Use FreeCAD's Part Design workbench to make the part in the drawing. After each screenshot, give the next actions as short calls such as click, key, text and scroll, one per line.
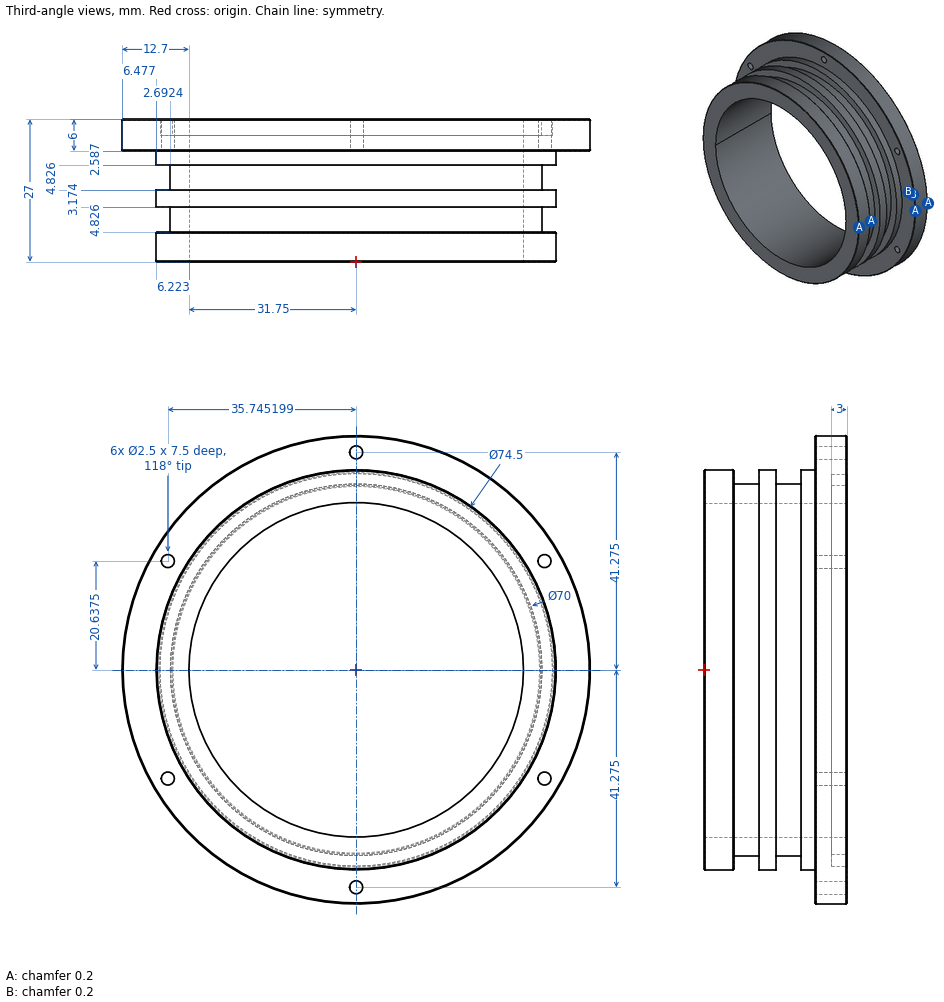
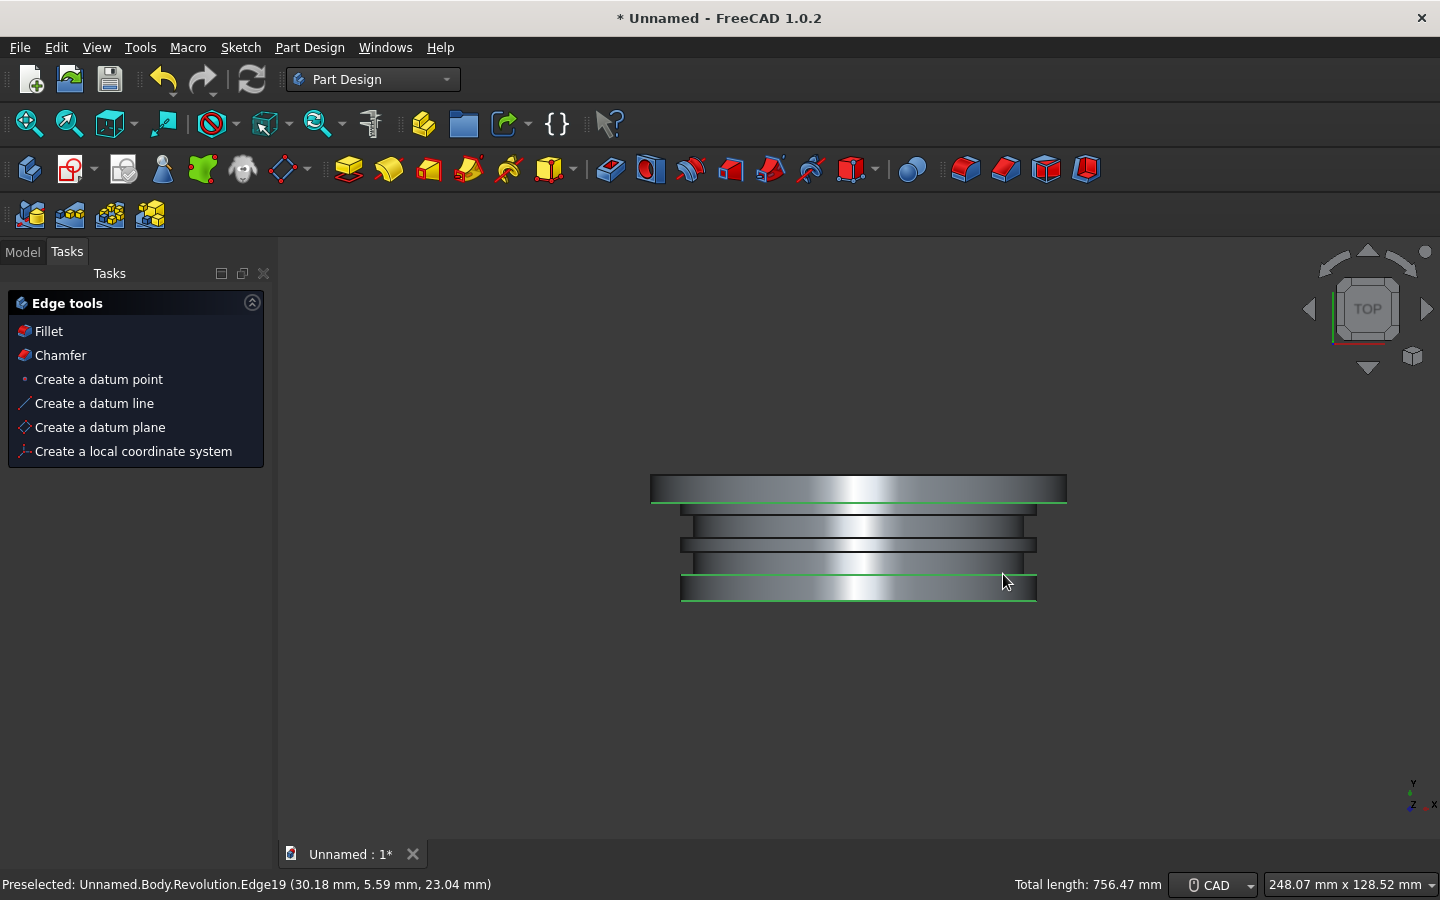
click(1028, 474, ctrl)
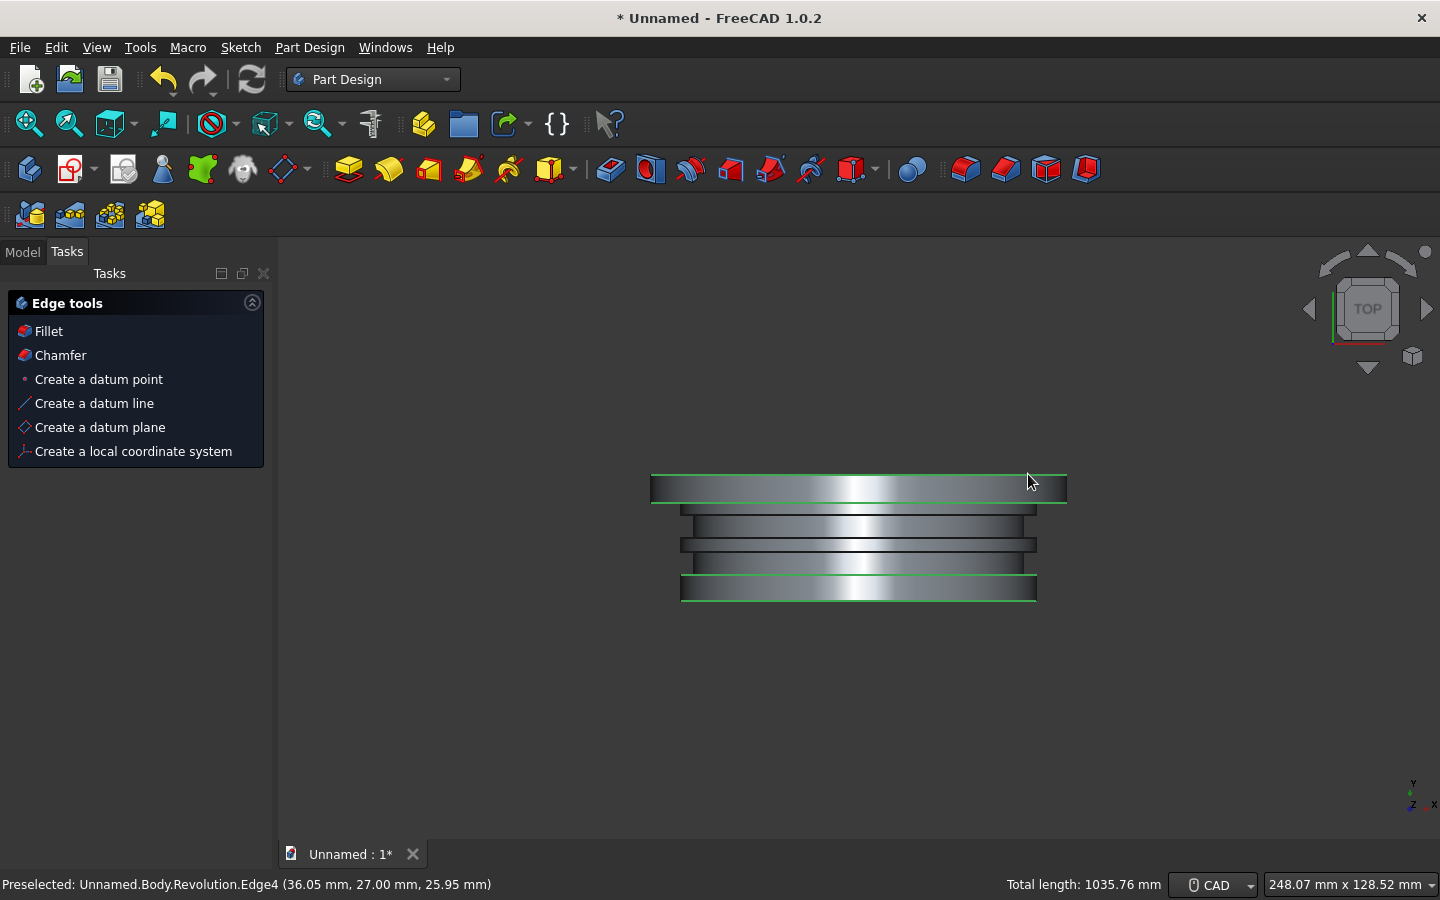
click(1006, 170)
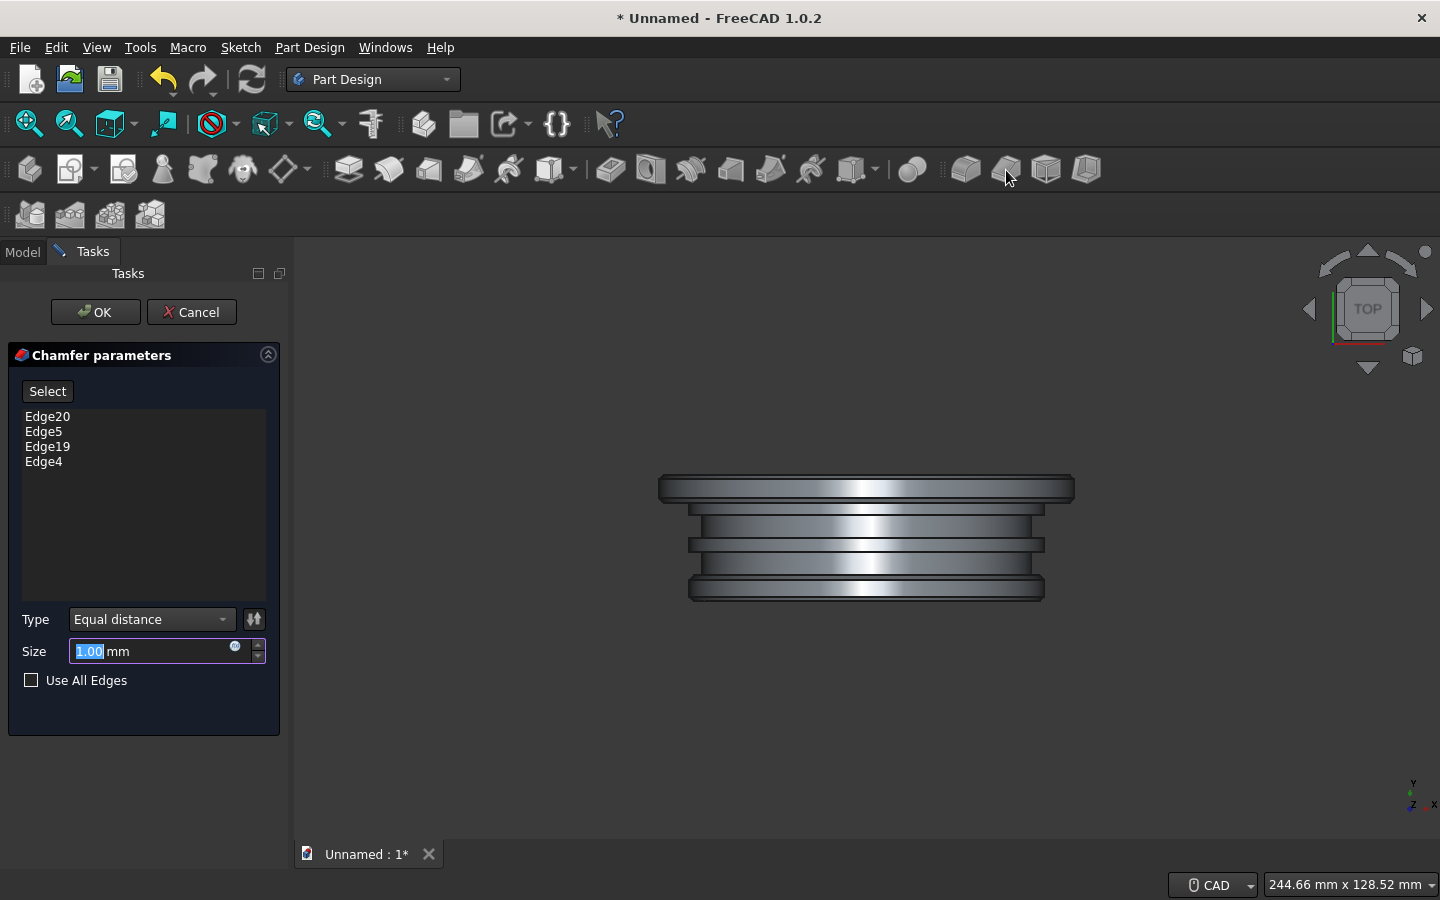
text(0.2)
key(Tab)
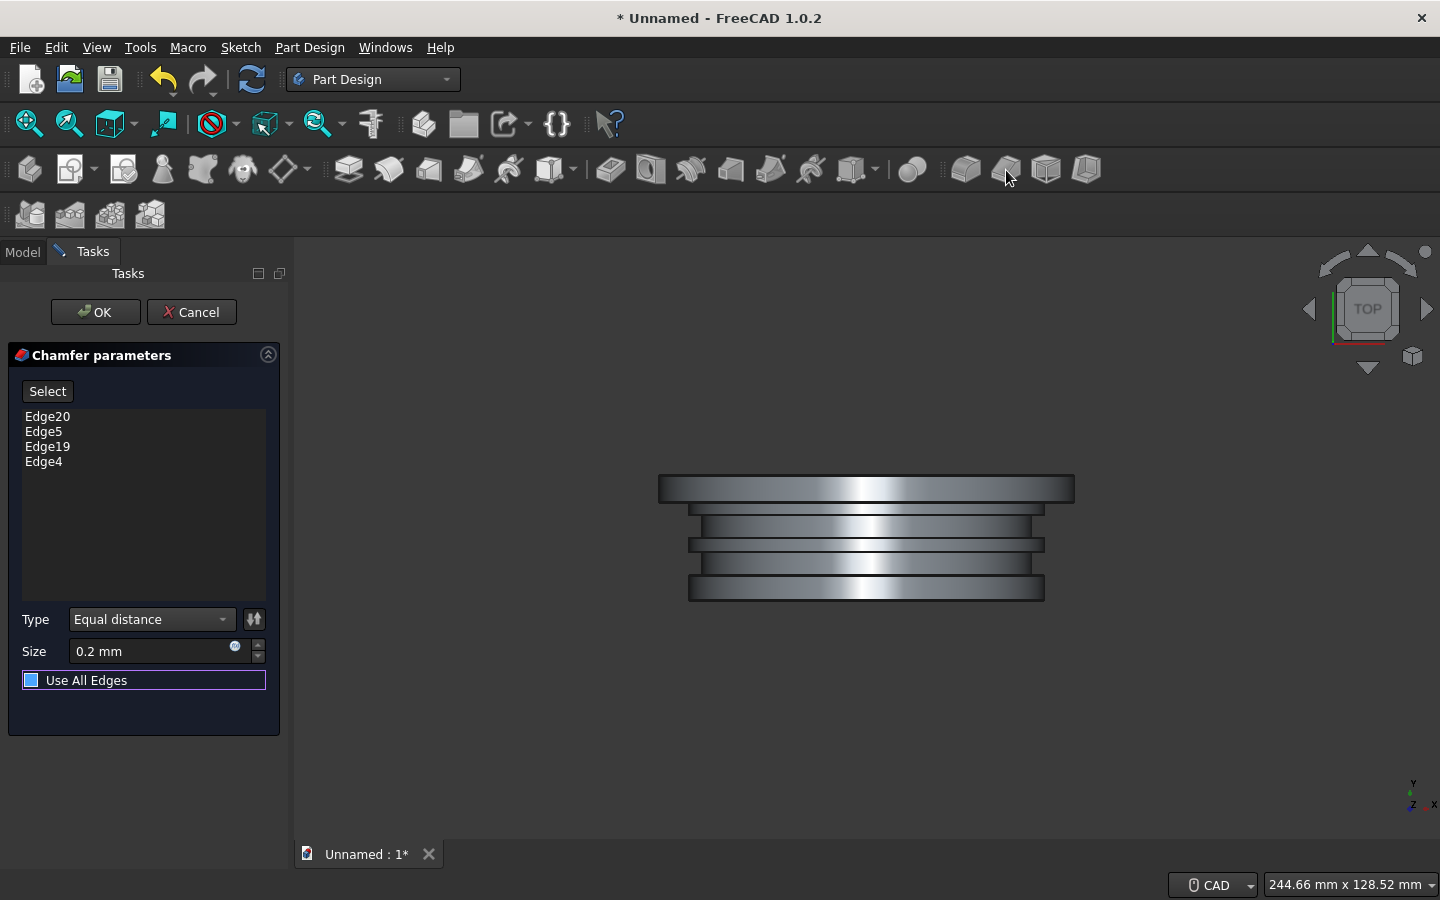
click(96, 312)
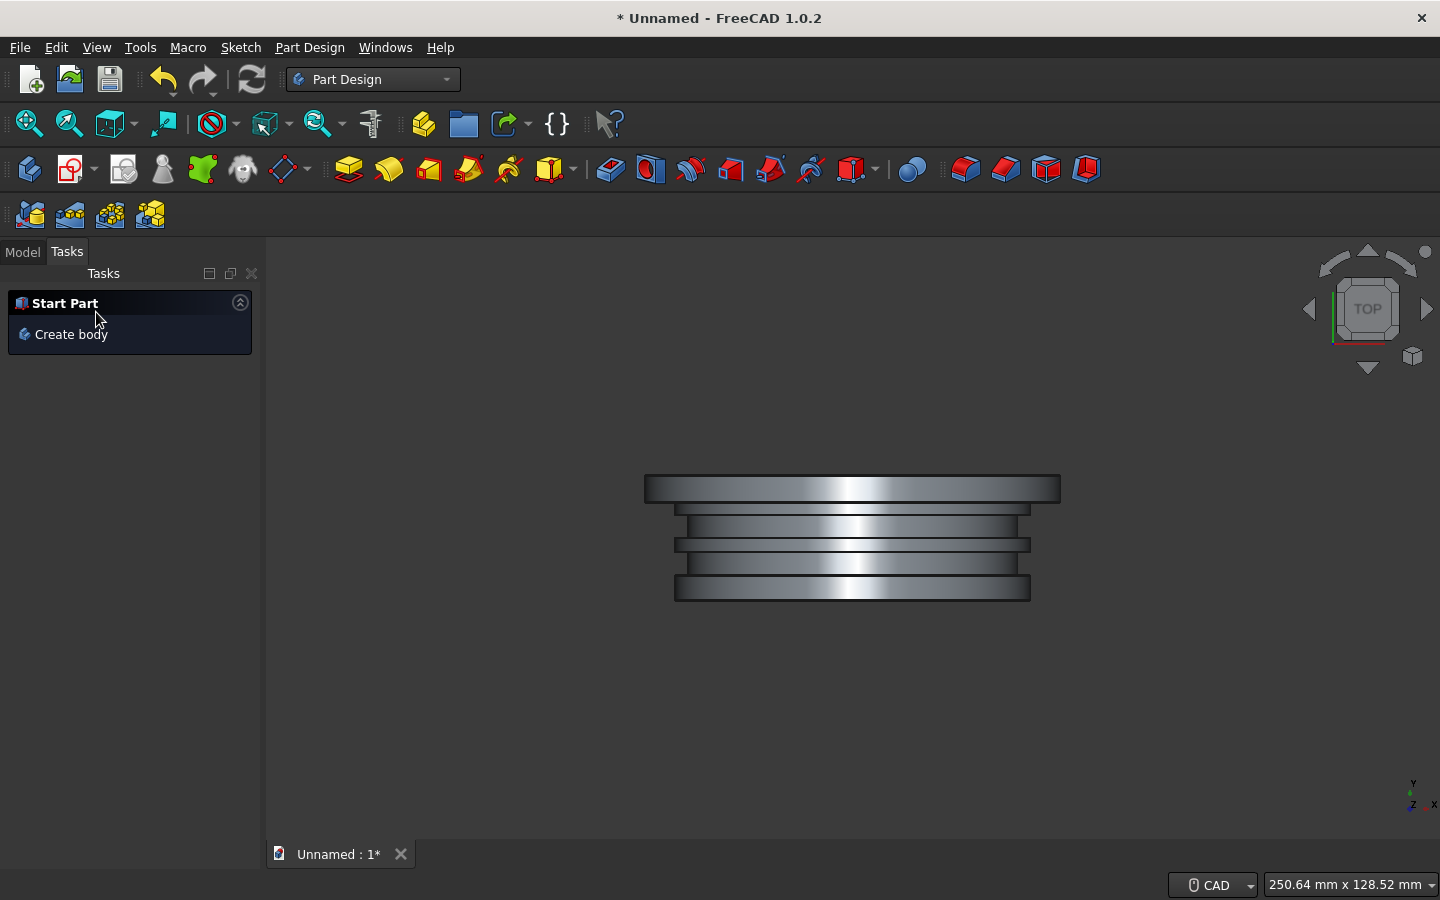
key(v)
key(f)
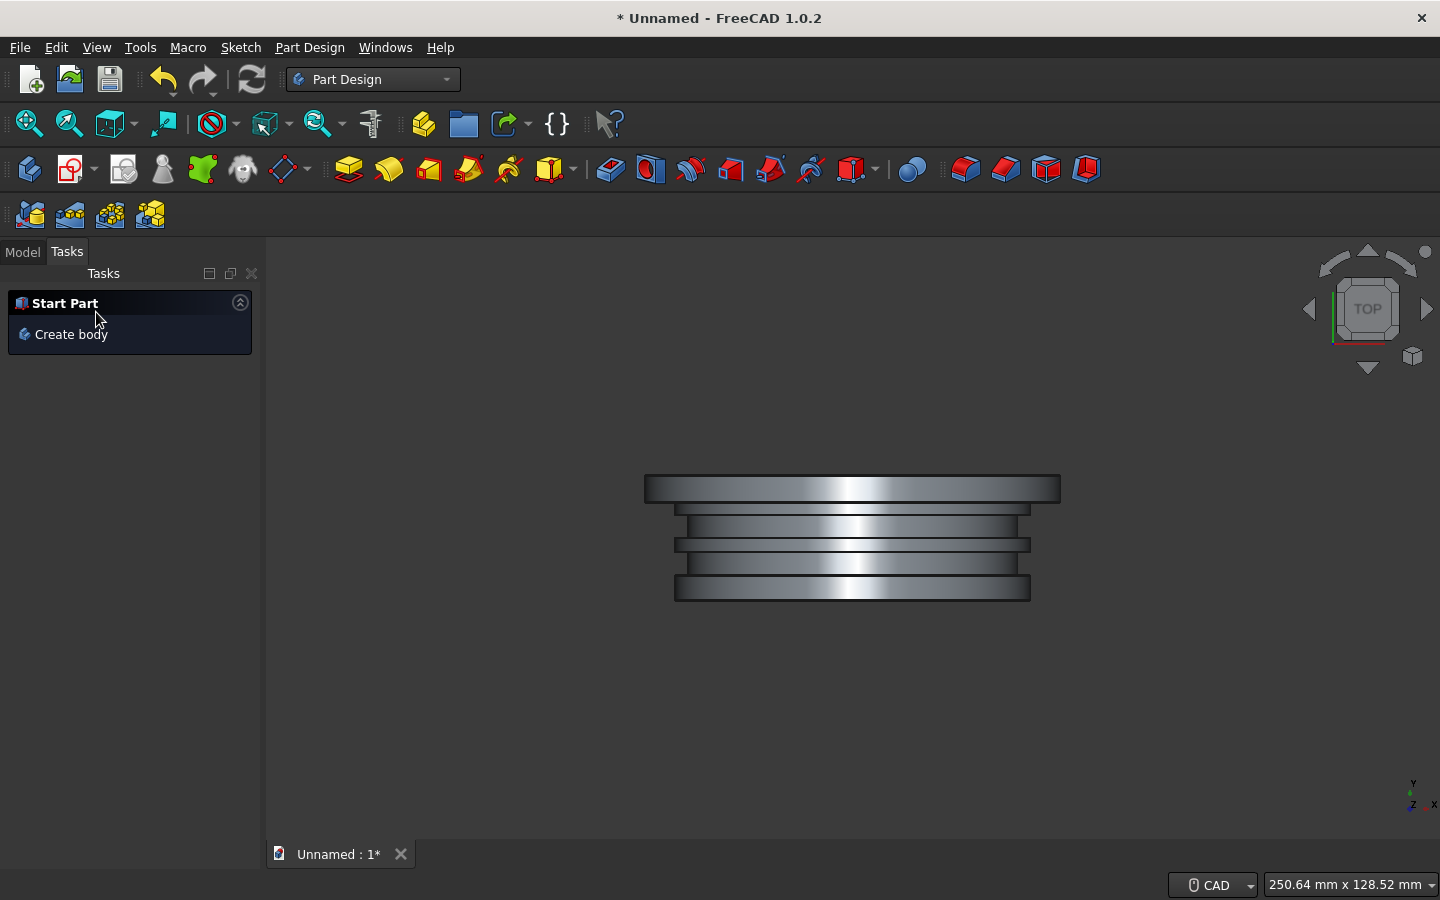
key(4)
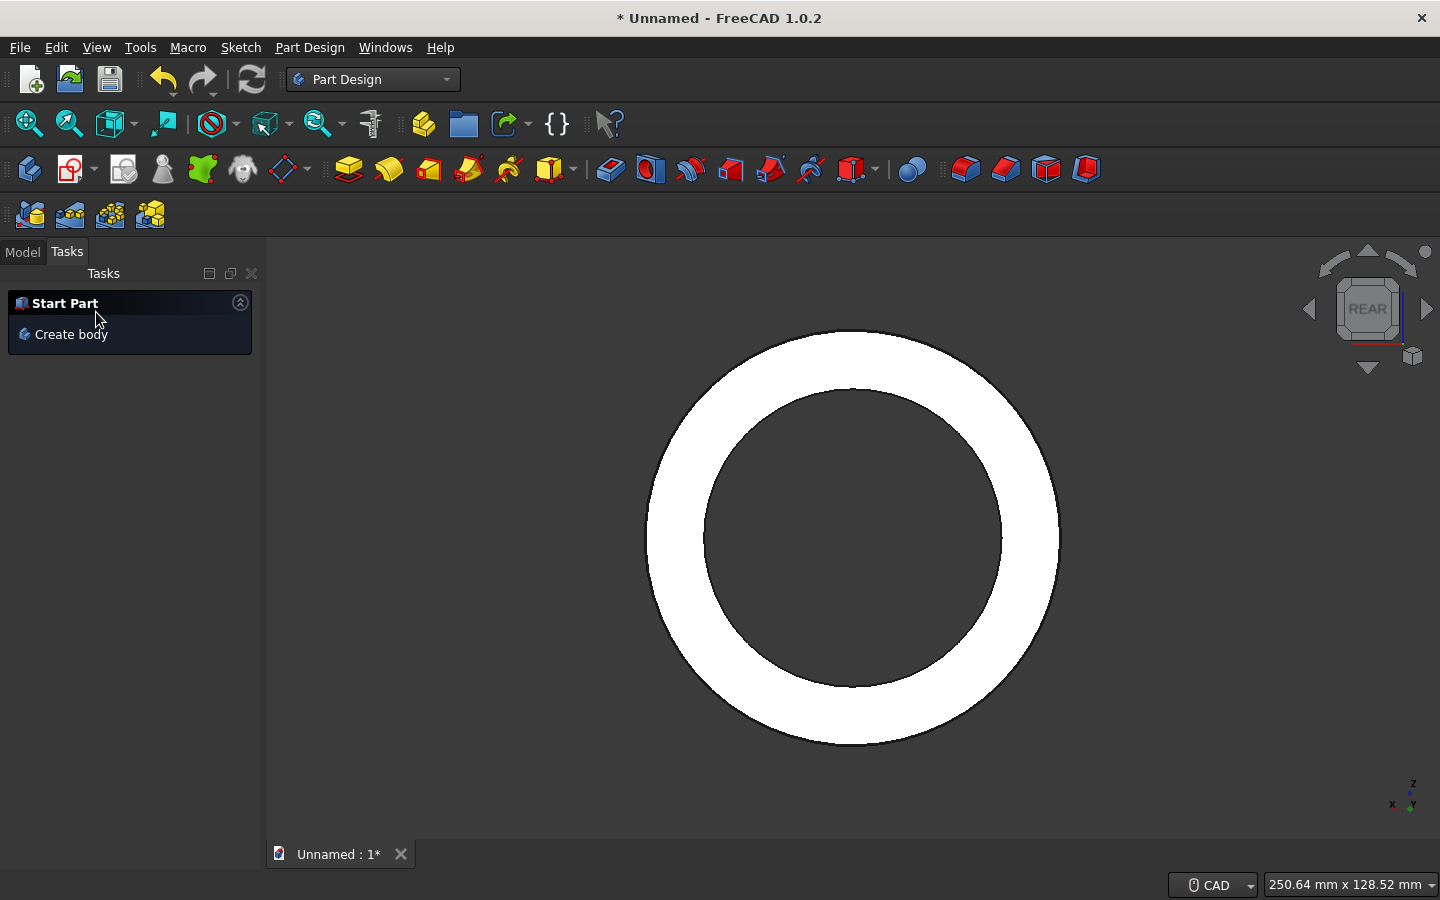
click(675, 537)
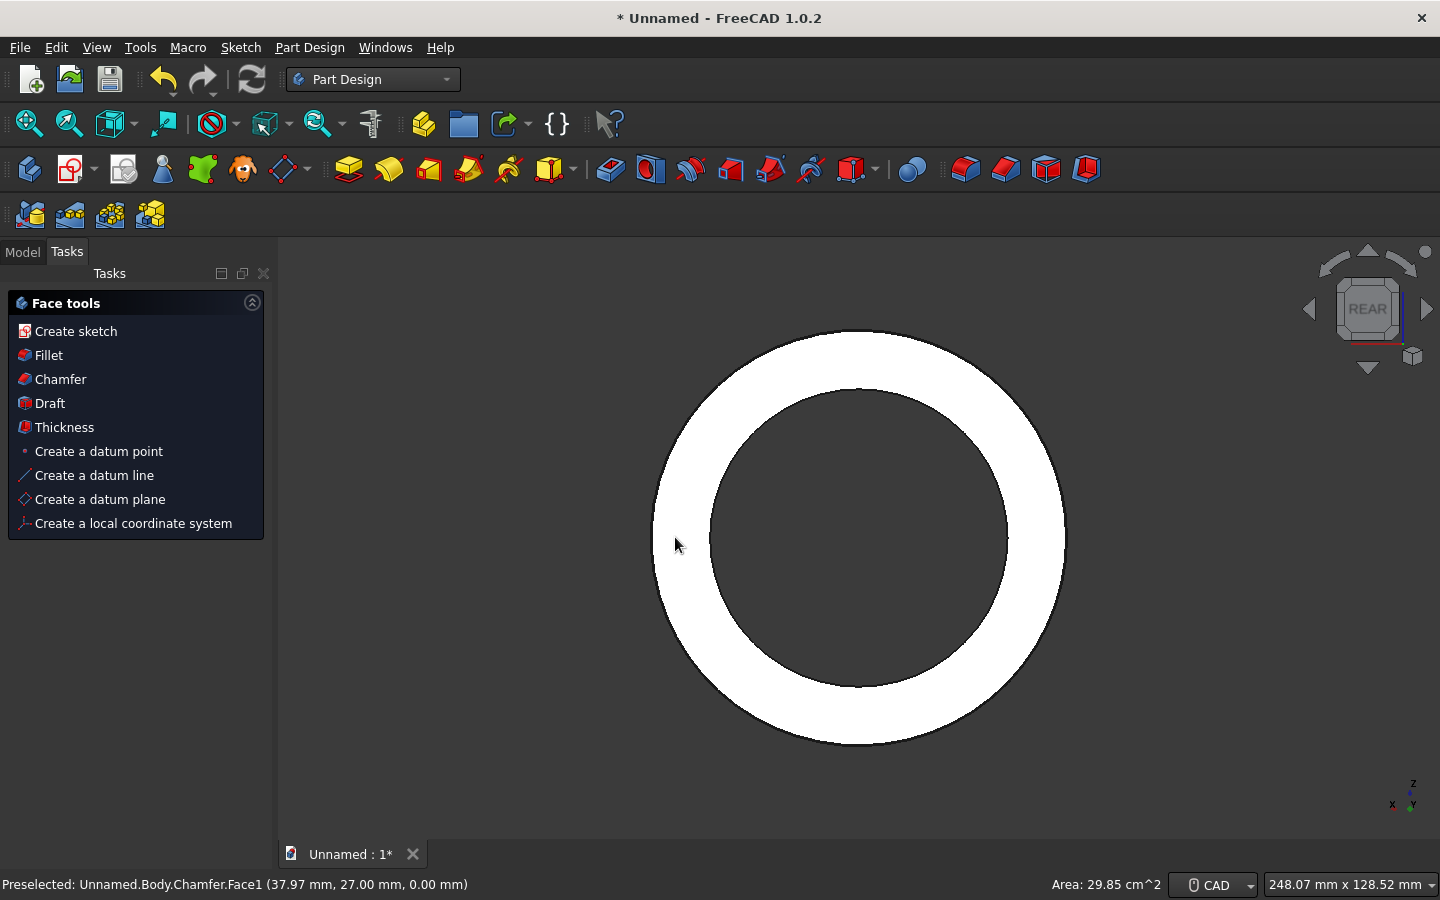
click(70, 170)